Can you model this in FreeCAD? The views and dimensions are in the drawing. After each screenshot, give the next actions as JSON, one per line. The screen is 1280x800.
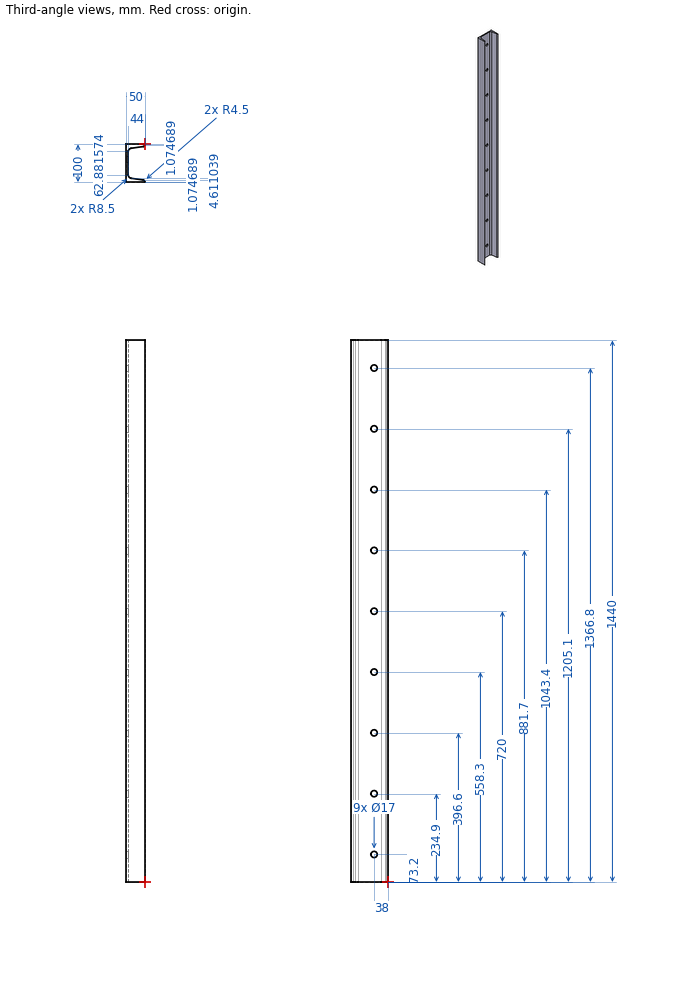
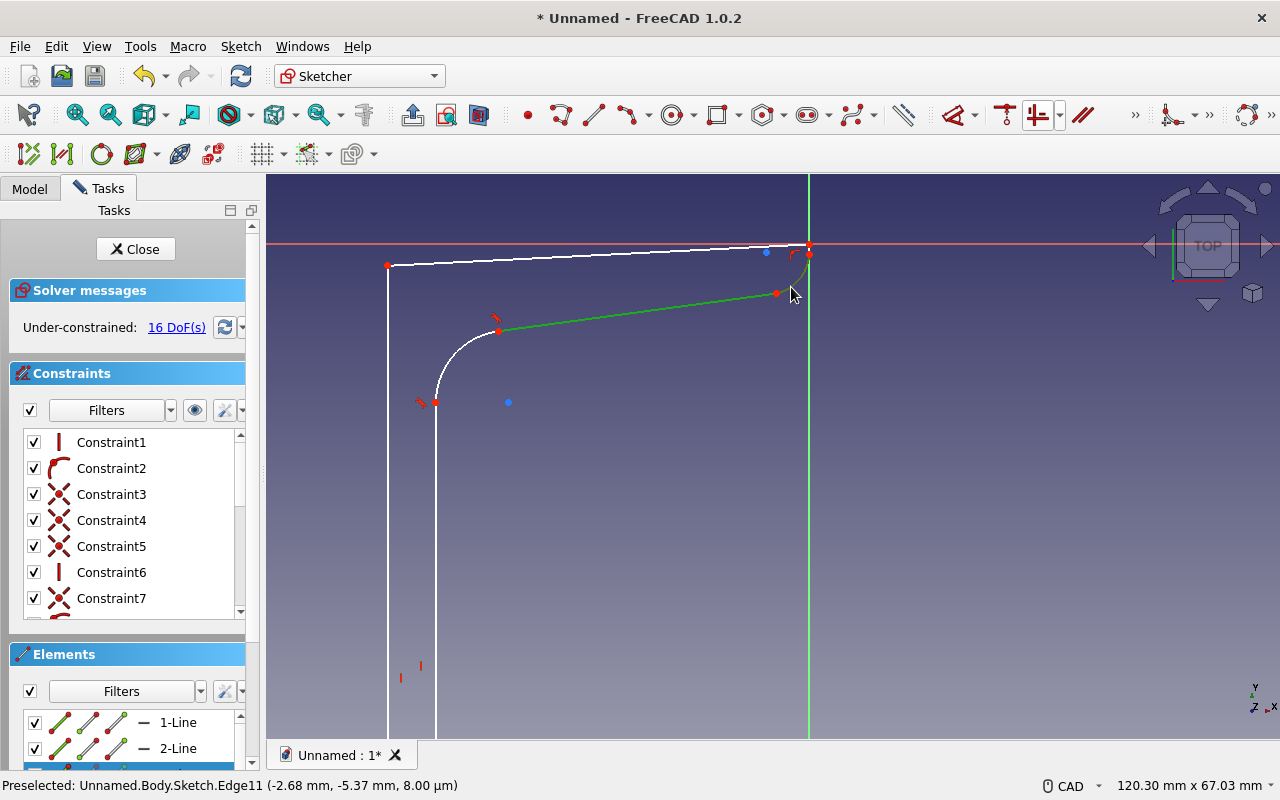
{"action": "key", "text": "t"}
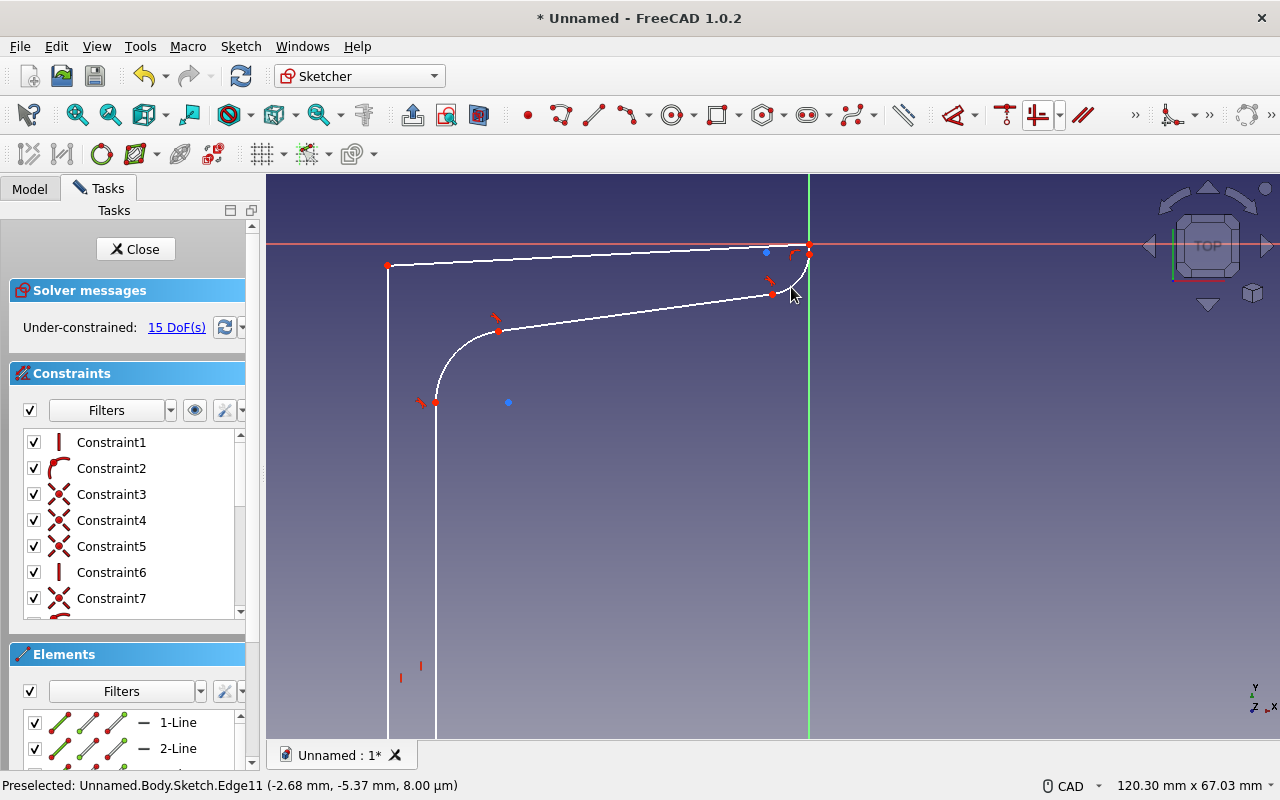
{"action": "scroll", "coordinate": [809, 249], "scroll_direction": "up", "scroll_amount": 6}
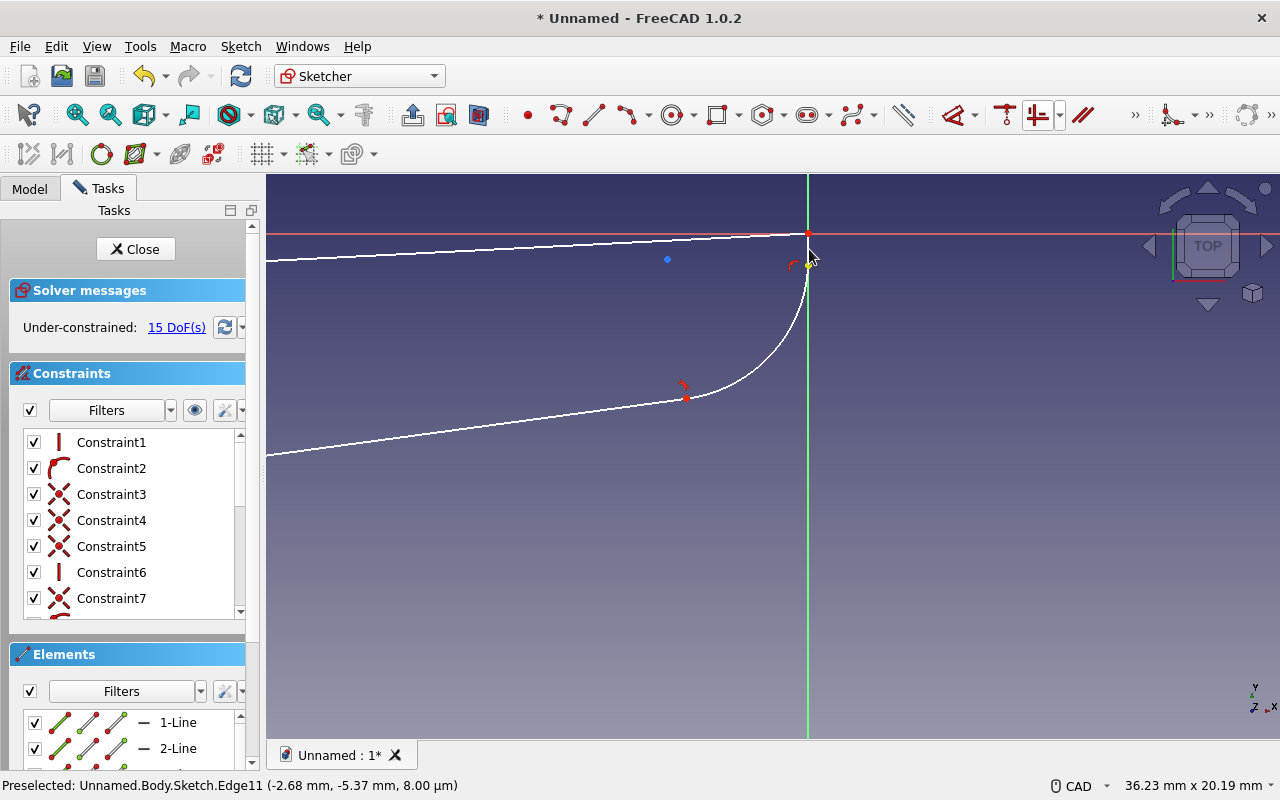
{"action": "left_click", "coordinate": [808, 250]}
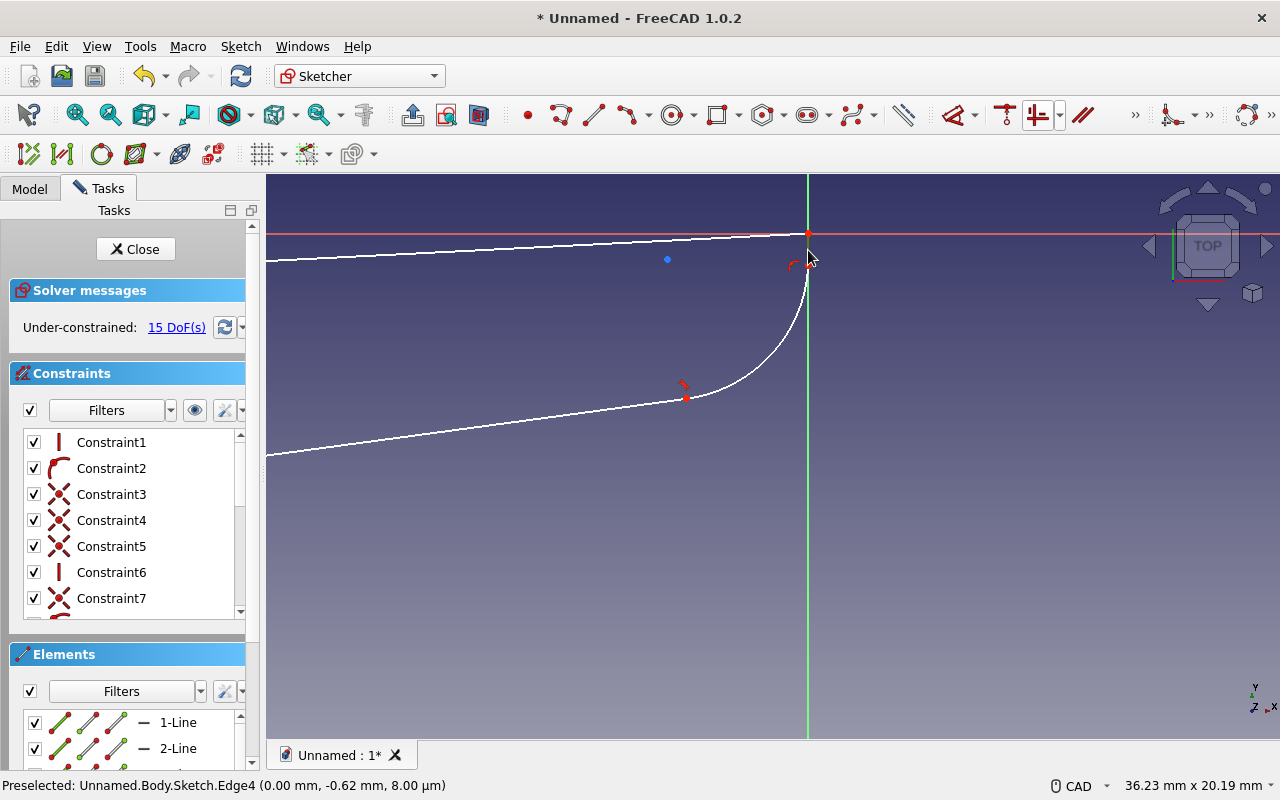
{"action": "scroll", "coordinate": [798, 272], "scroll_direction": "down", "scroll_amount": 10}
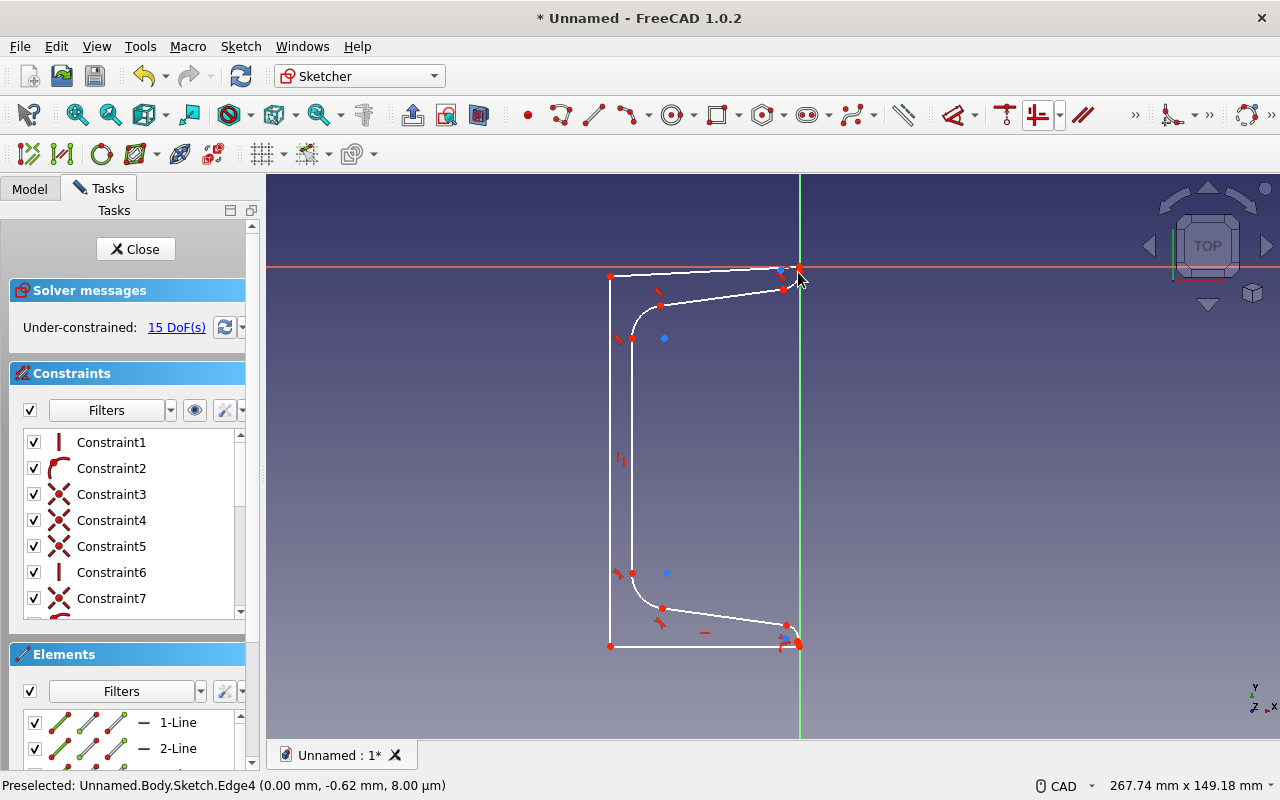
{"action": "scroll", "coordinate": [791, 287], "scroll_direction": "up", "scroll_amount": 3}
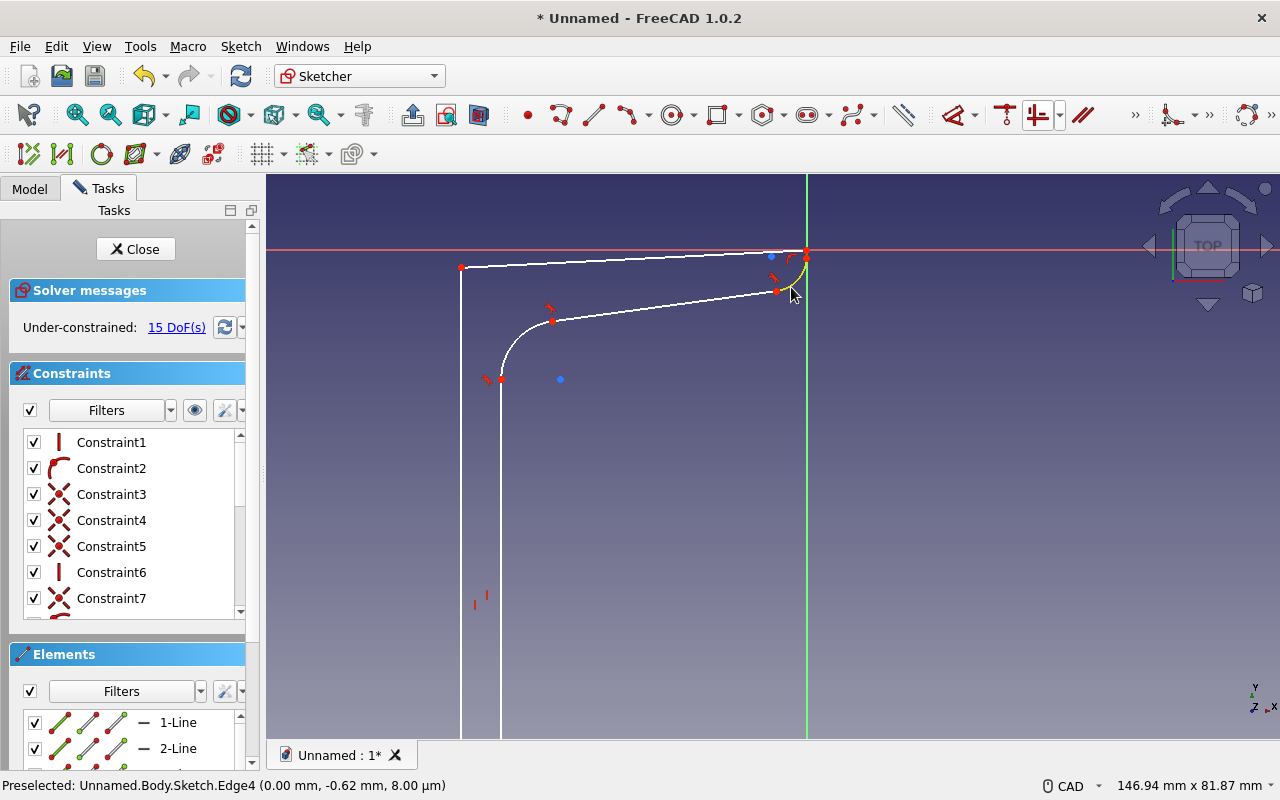
{"action": "left_click", "coordinate": [790, 286]}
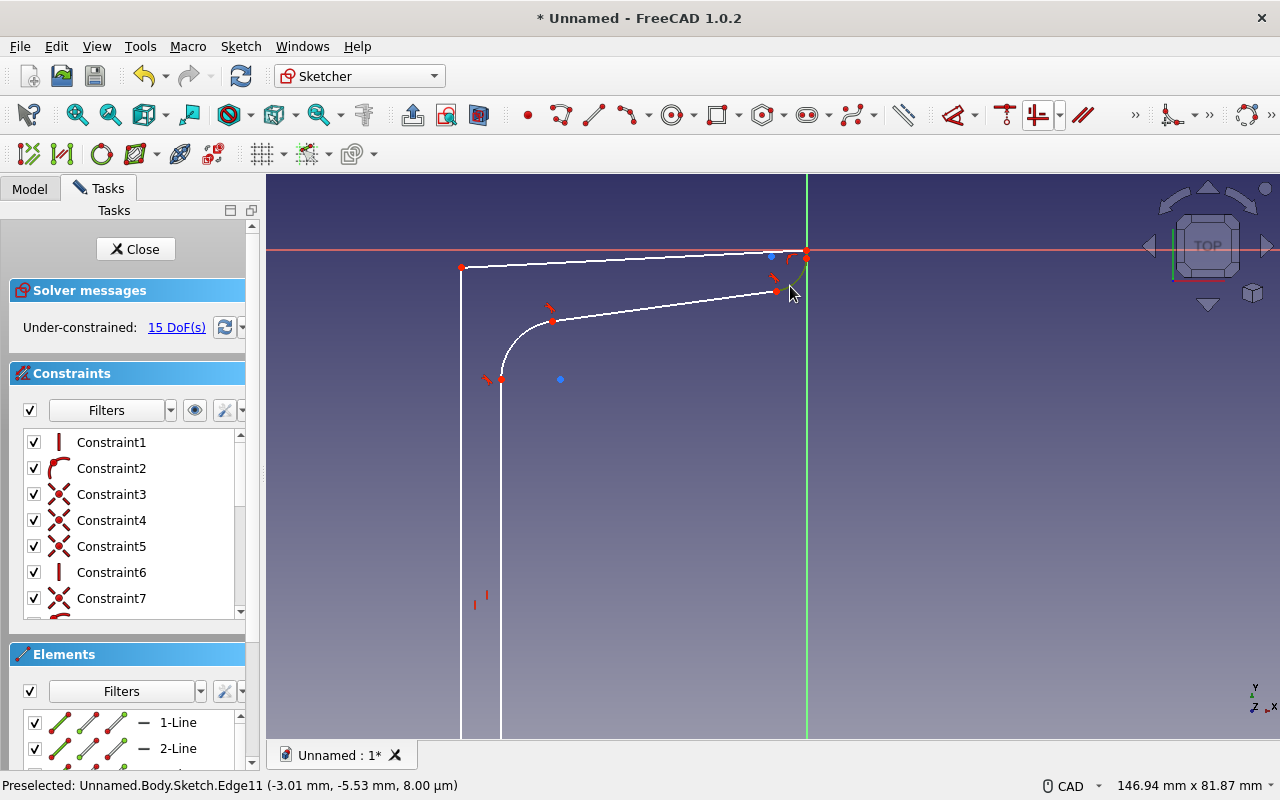
{"action": "key", "text": "t"}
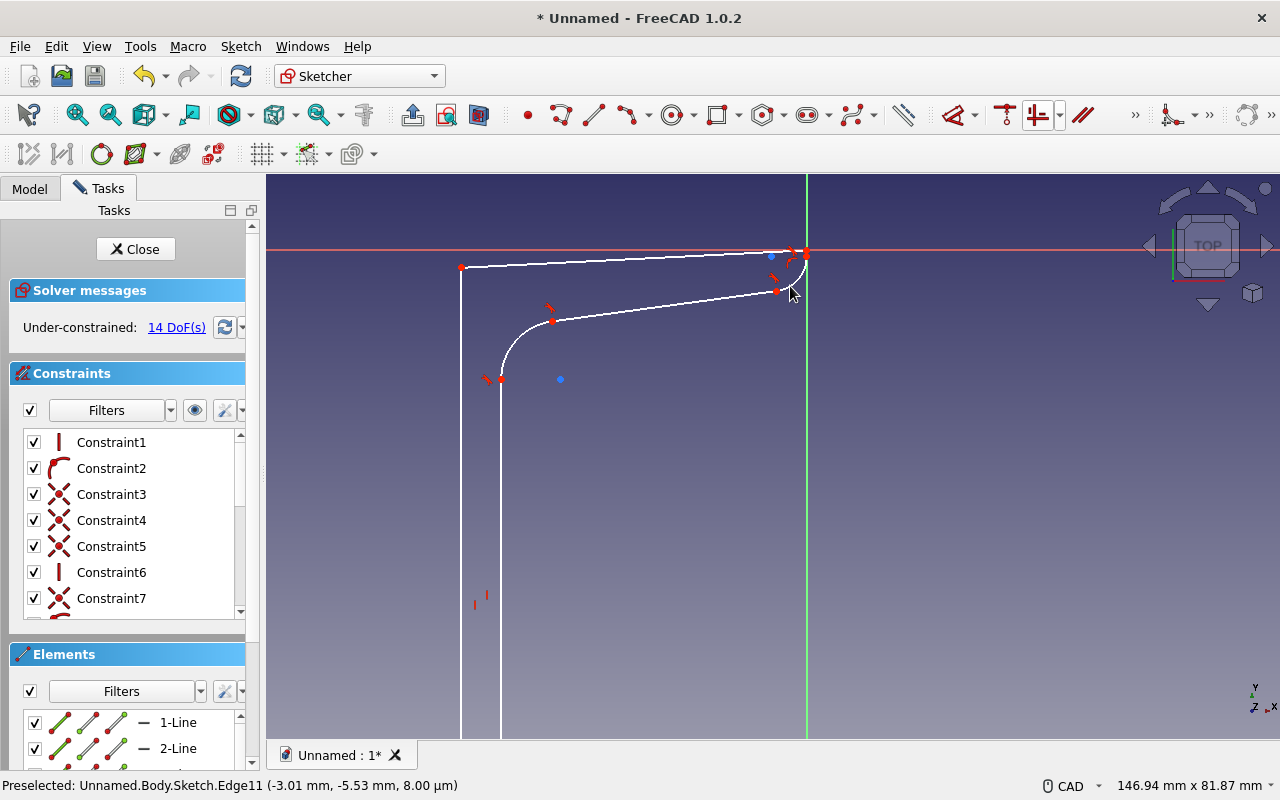
{"action": "scroll", "coordinate": [790, 288], "scroll_direction": "down", "scroll_amount": 3}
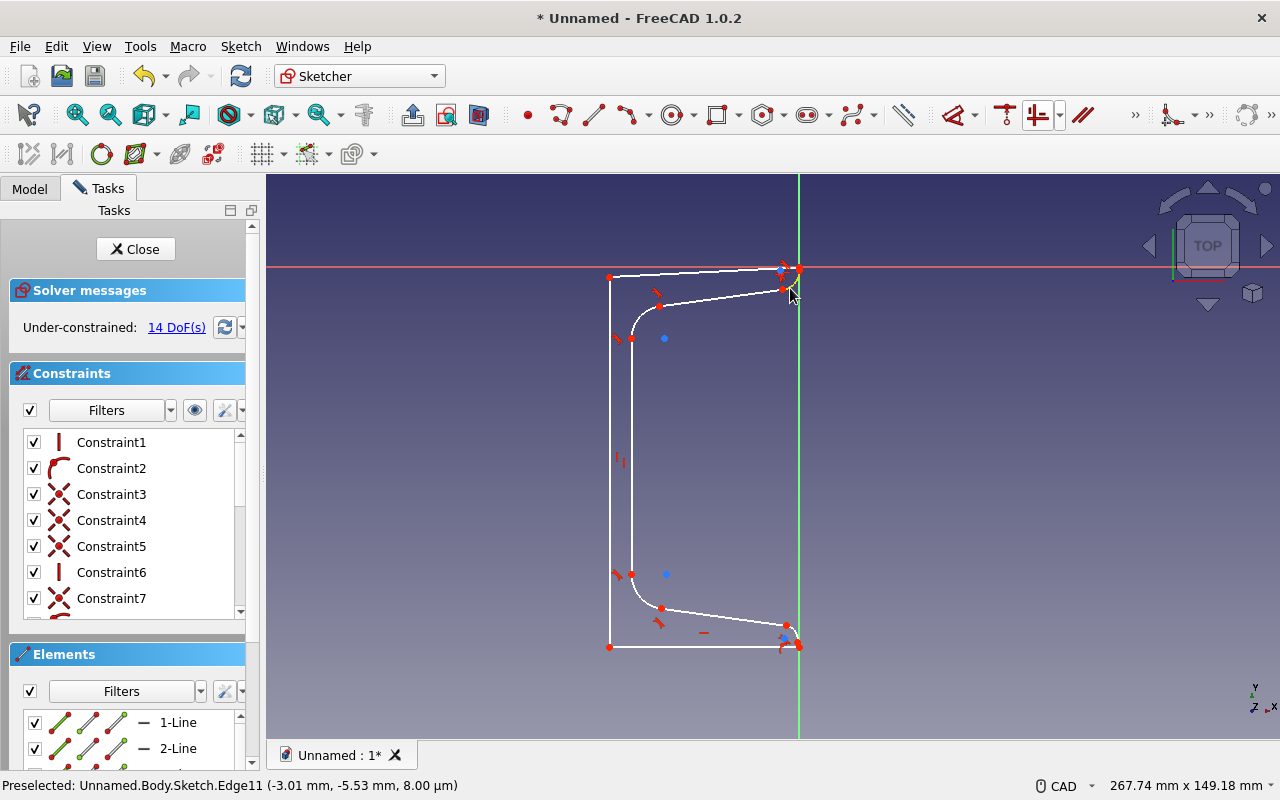
{"action": "scroll", "coordinate": [798, 645], "scroll_direction": "up", "scroll_amount": 9}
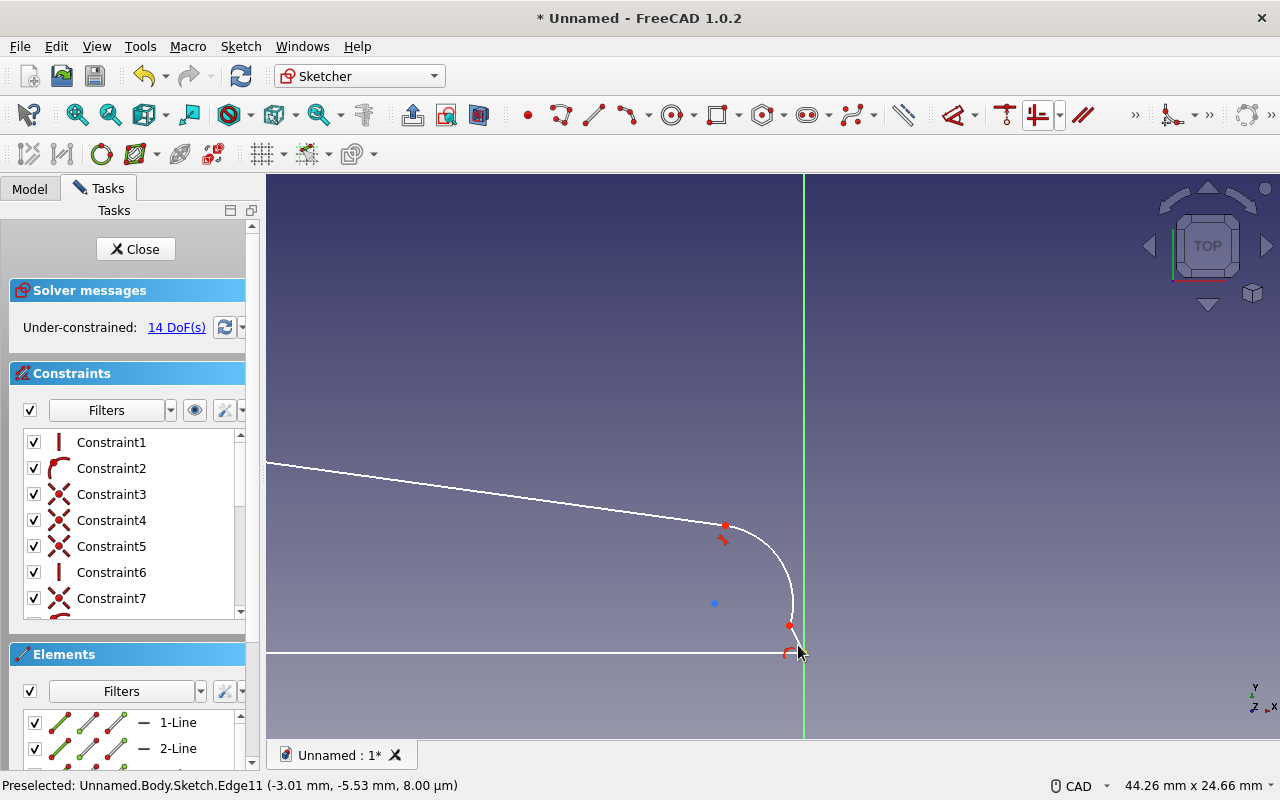
{"action": "left_click", "coordinate": [797, 639]}